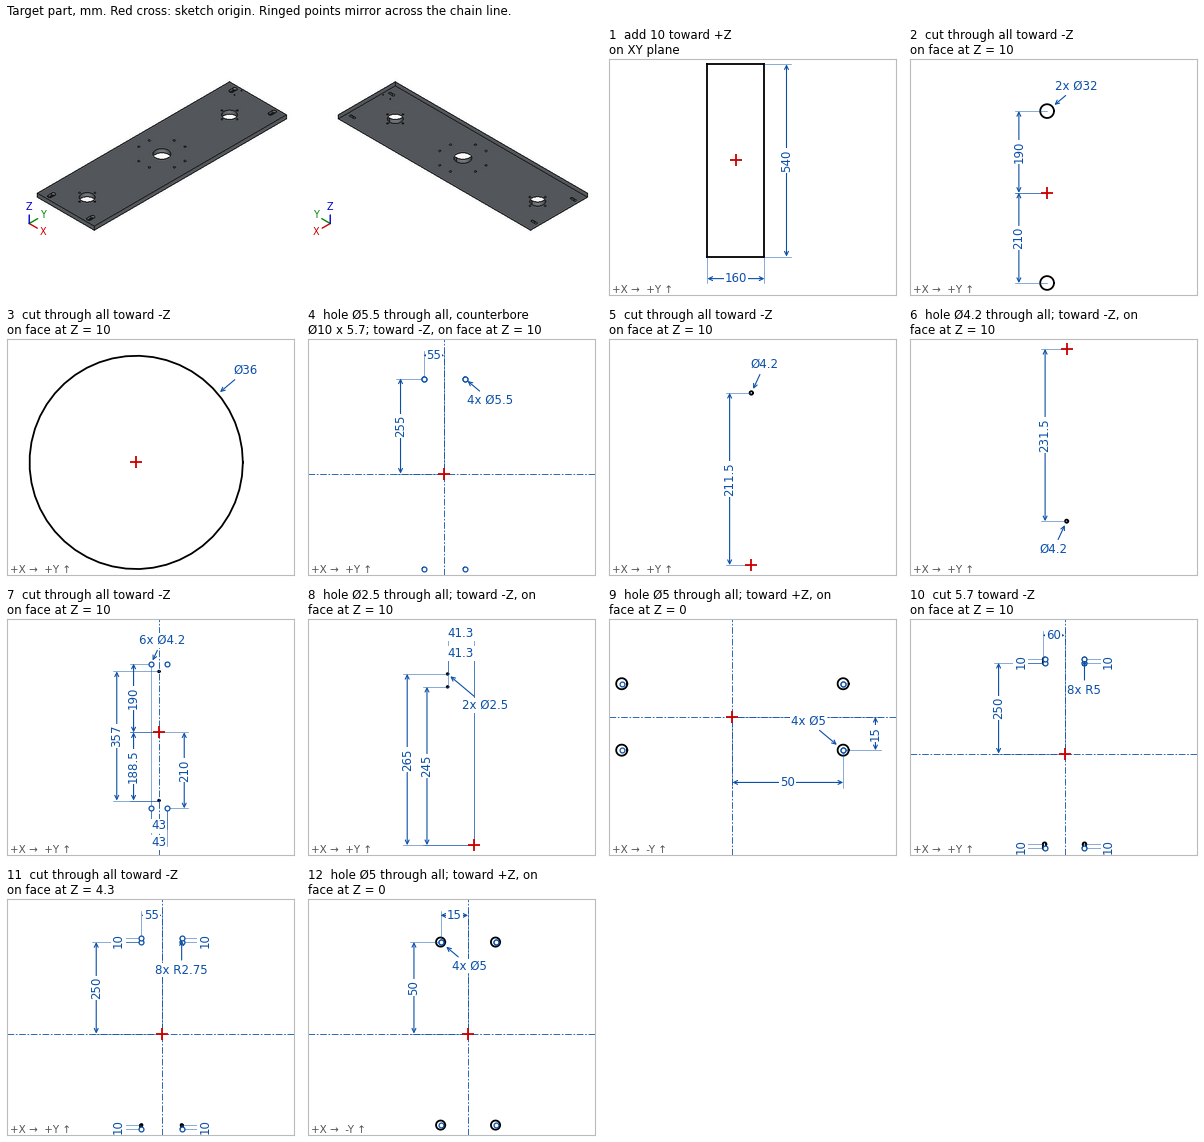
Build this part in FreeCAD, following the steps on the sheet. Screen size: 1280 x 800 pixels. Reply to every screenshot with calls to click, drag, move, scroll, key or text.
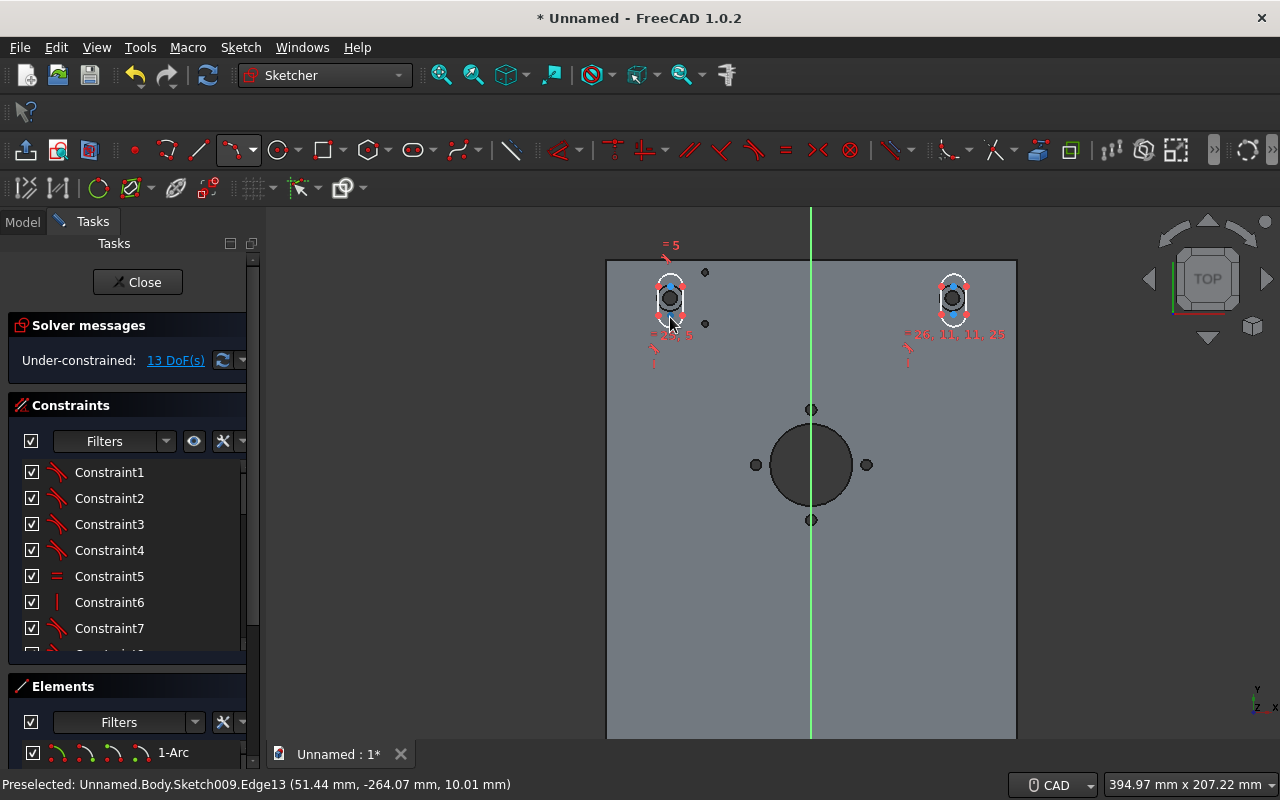
click(671, 315)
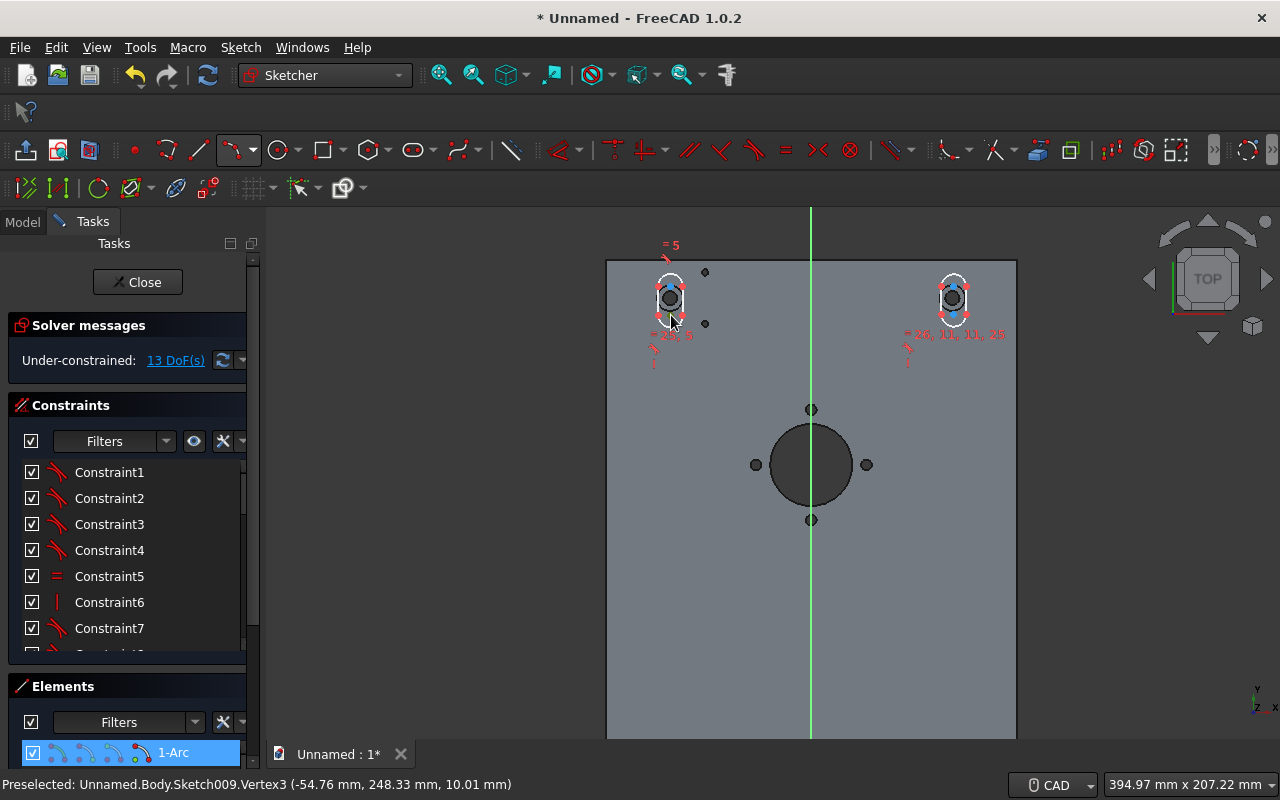
click(954, 314)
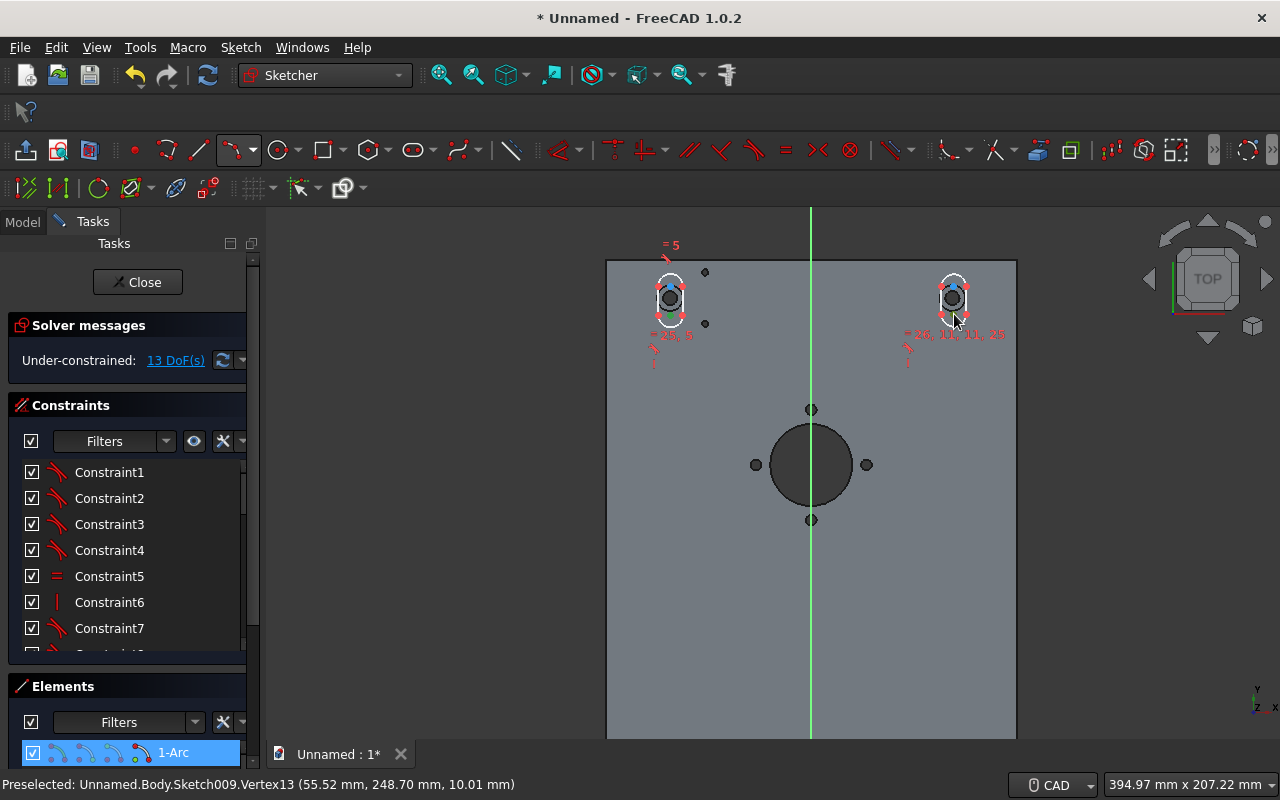
click(811, 677)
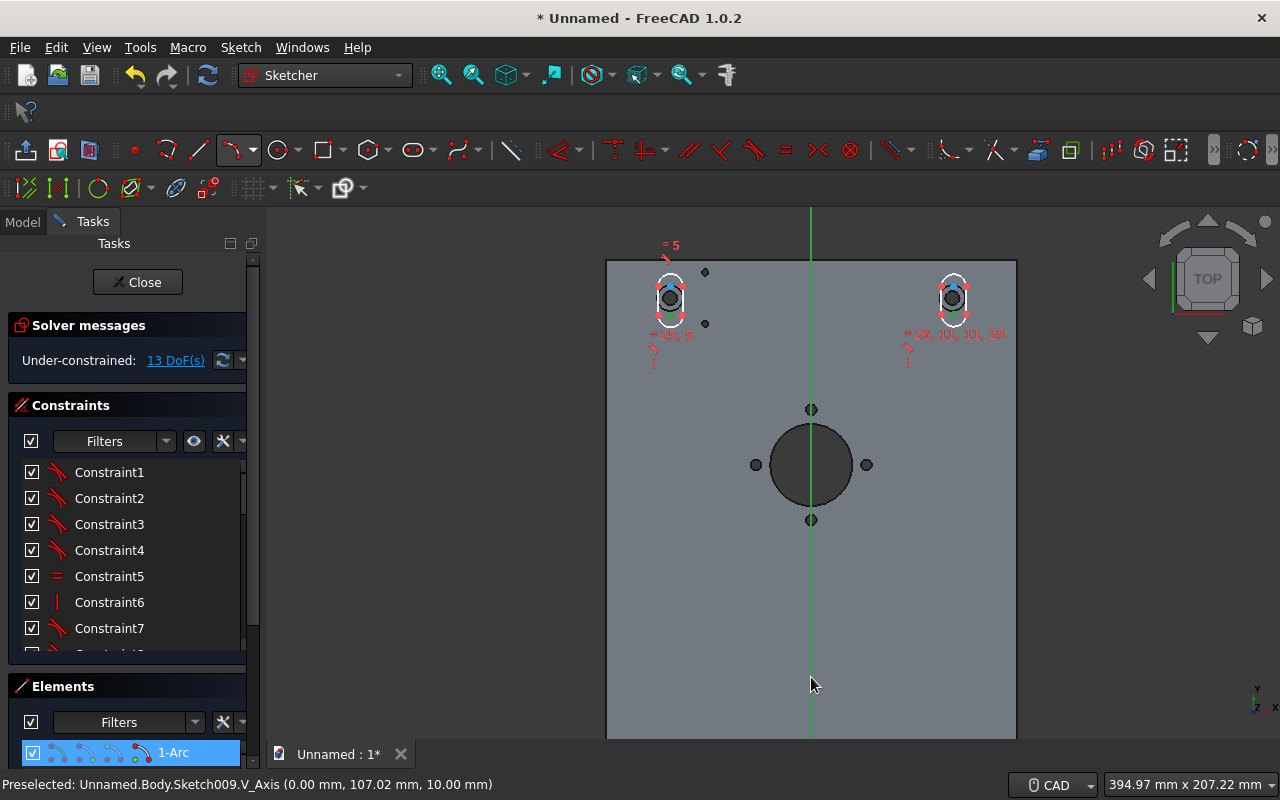
click(818, 150)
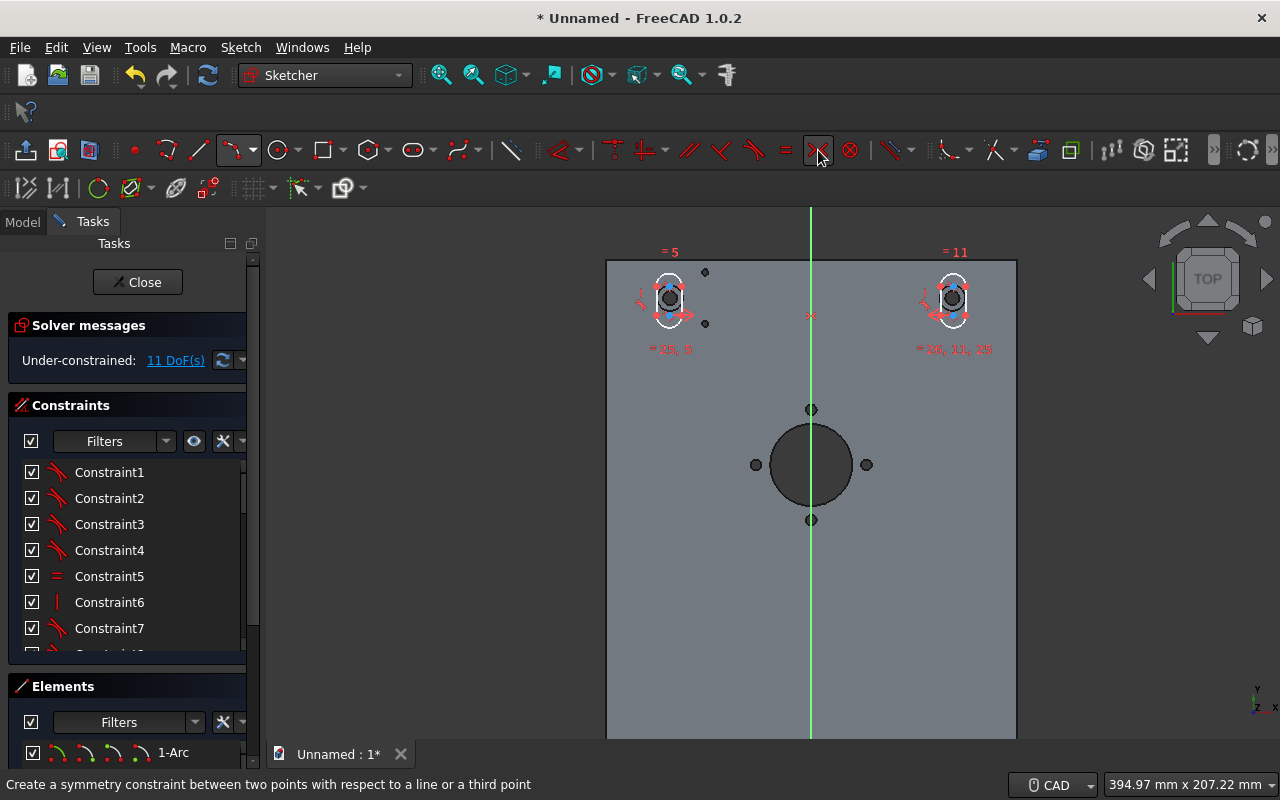
click(669, 286)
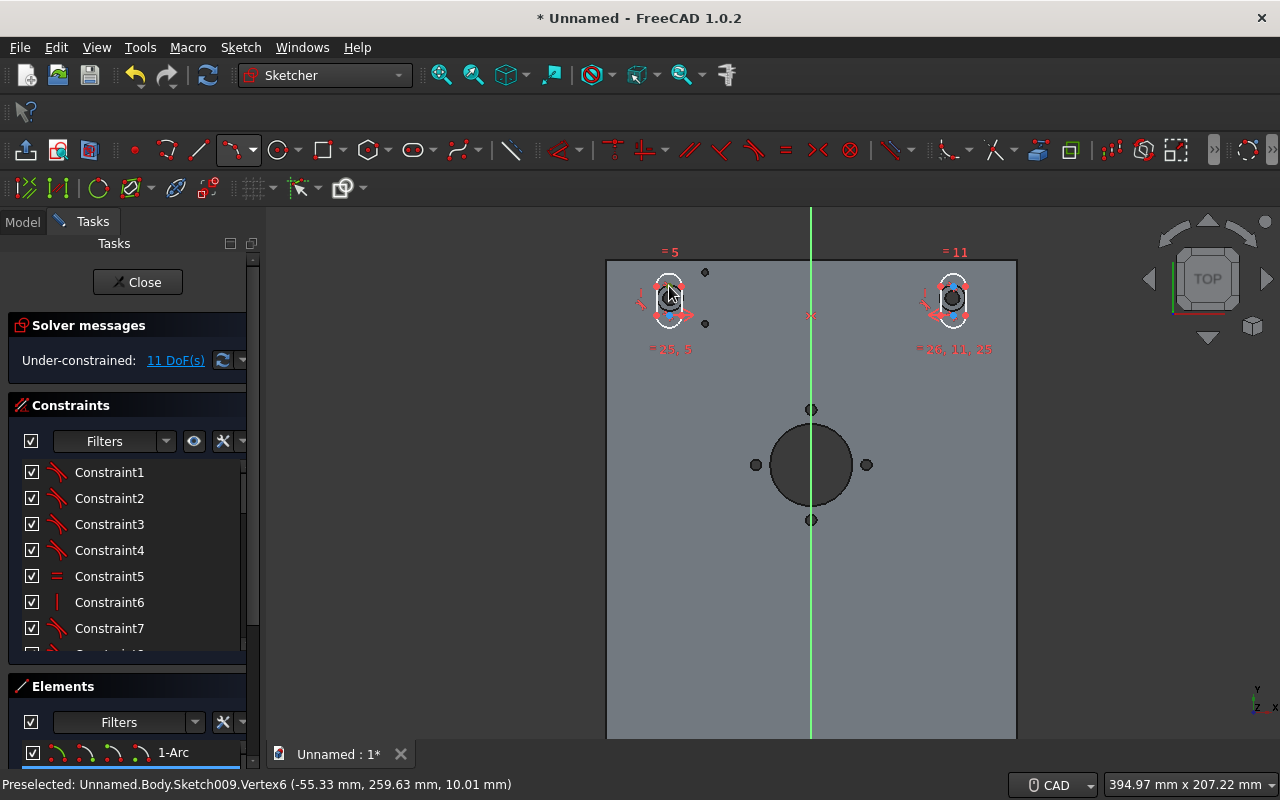
scroll(670, 316, down, 7)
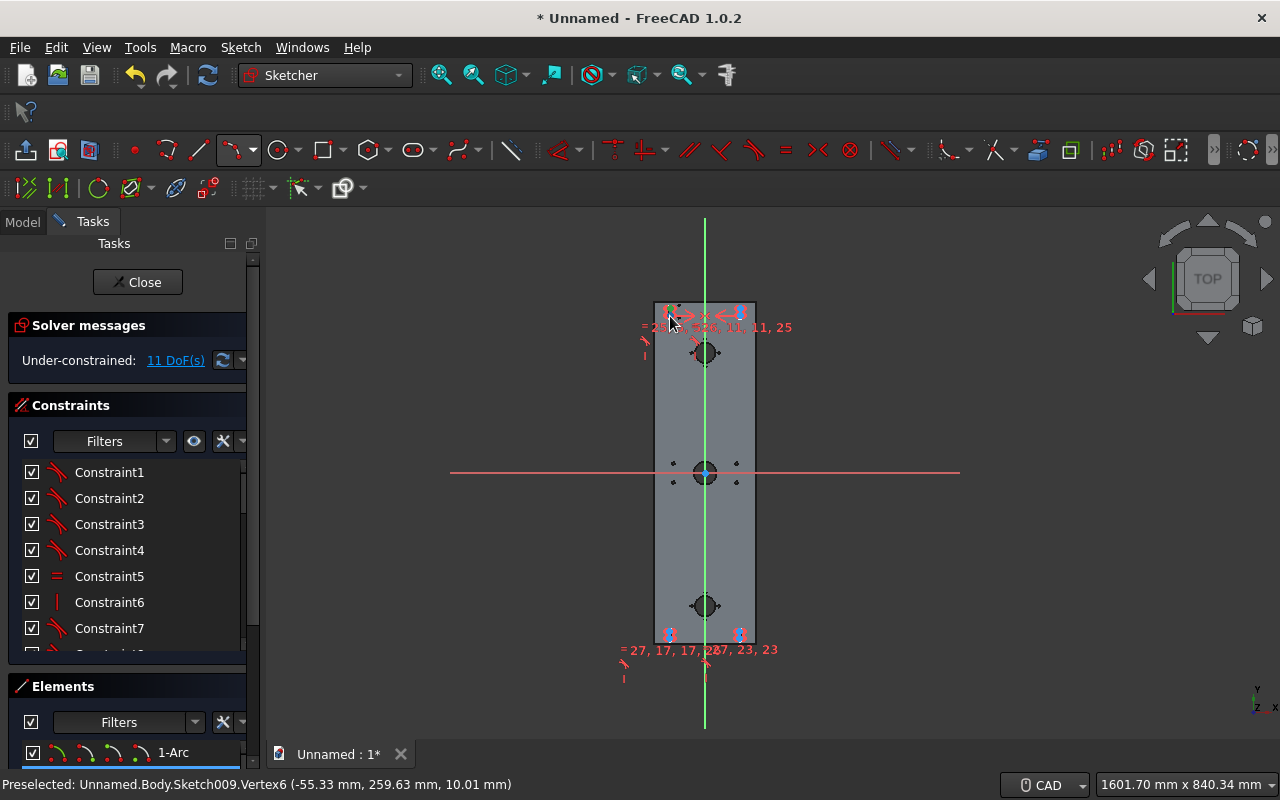
scroll(670, 639, up, 7)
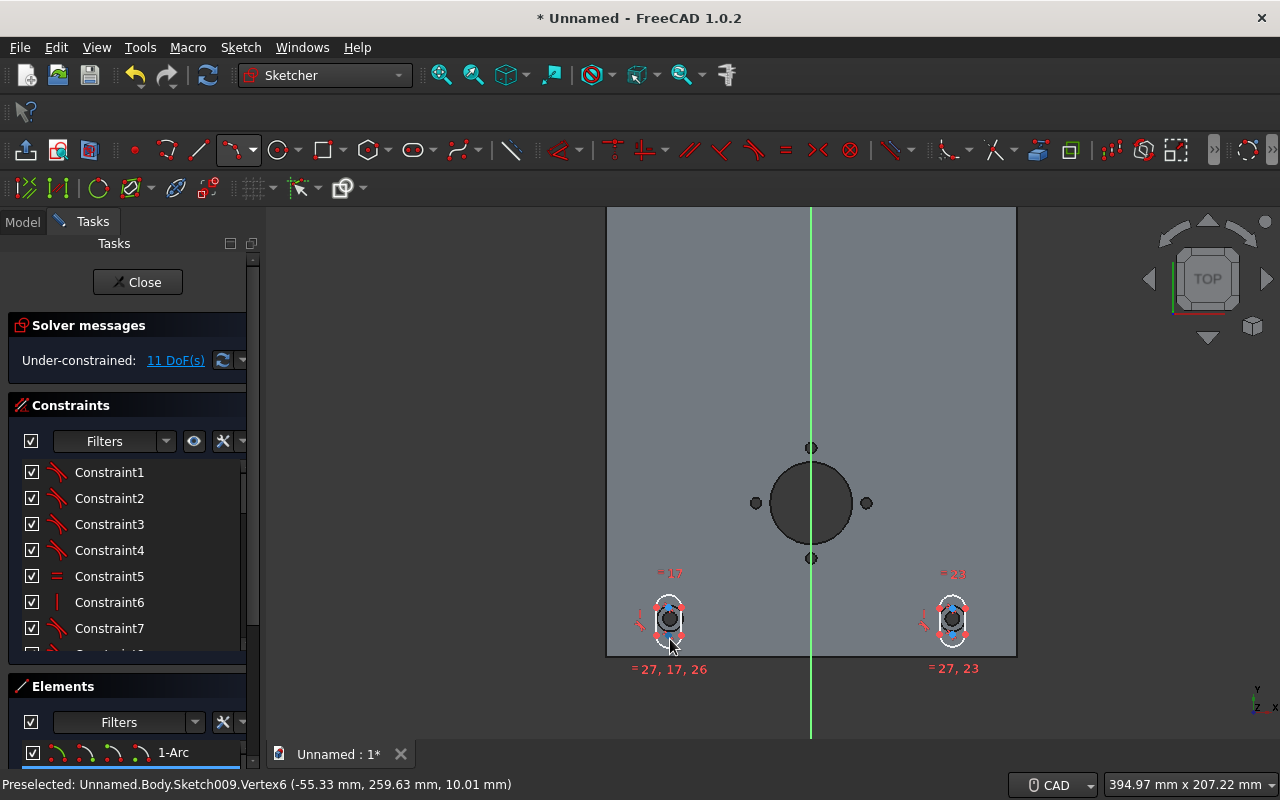
click(669, 635)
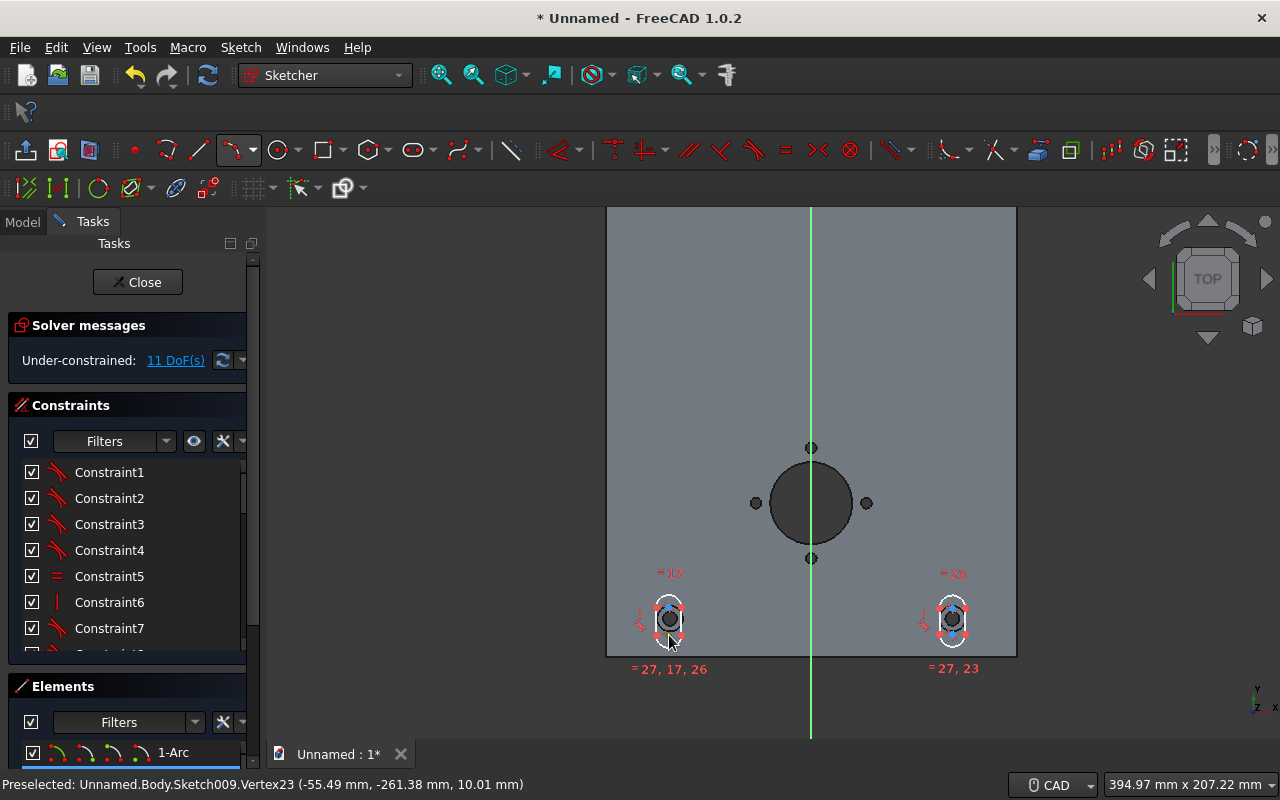
scroll(670, 640, down, 7)